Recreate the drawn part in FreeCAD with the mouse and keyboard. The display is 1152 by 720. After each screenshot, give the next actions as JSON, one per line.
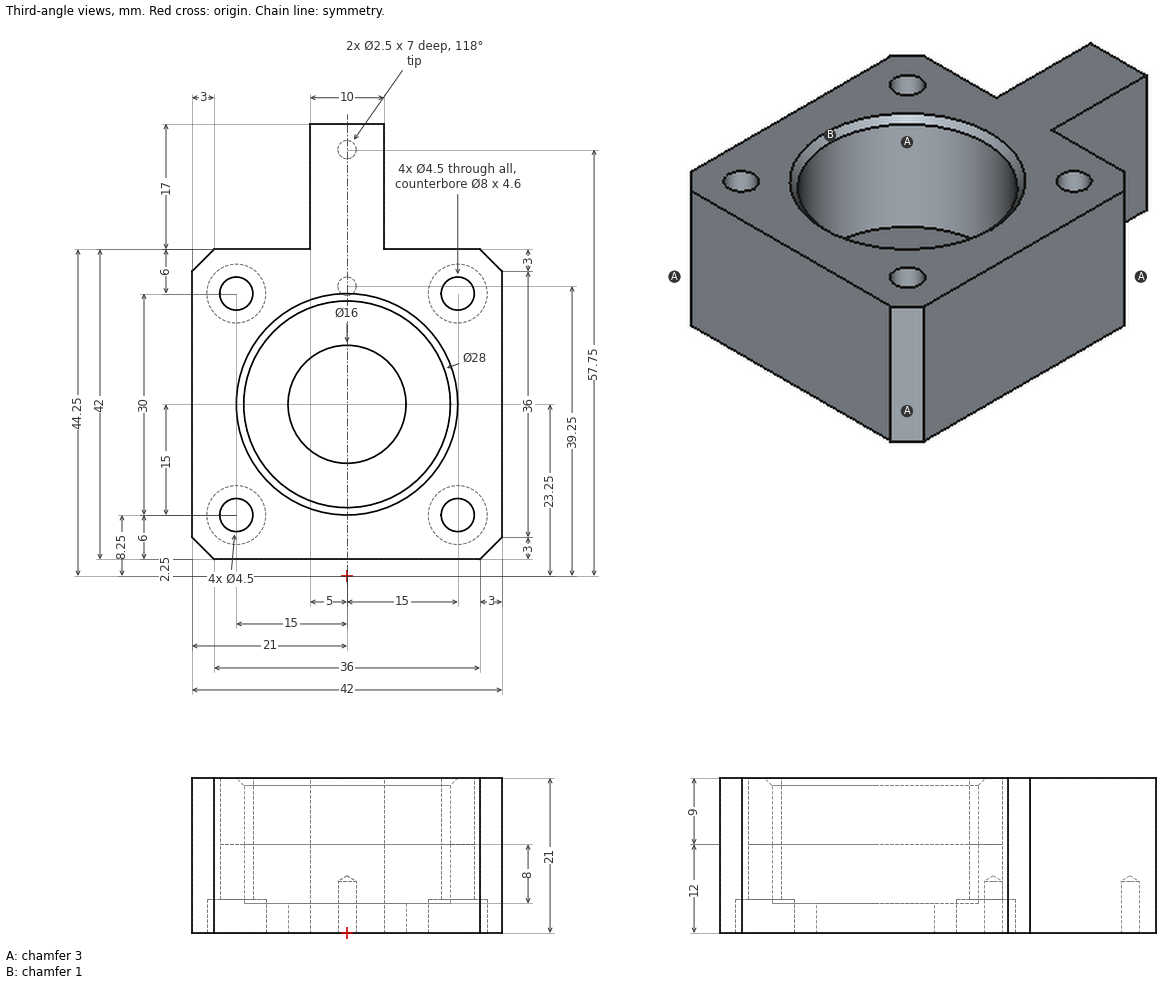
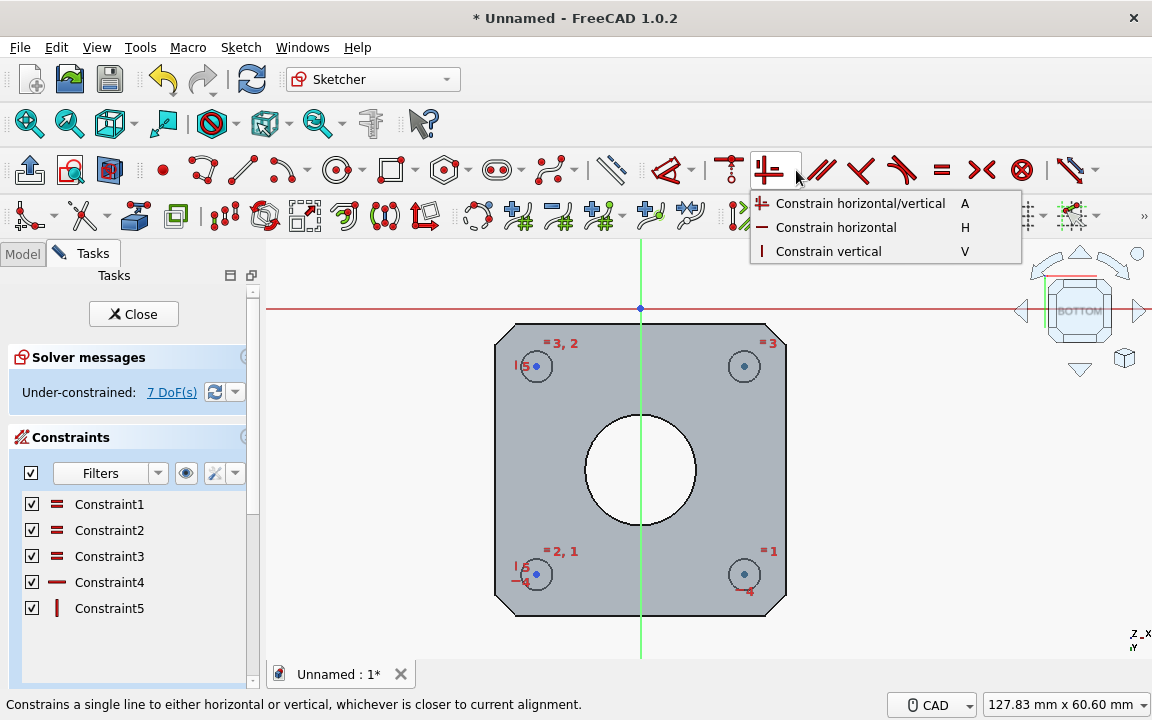
{"action": "left_click", "coordinate": [886, 251]}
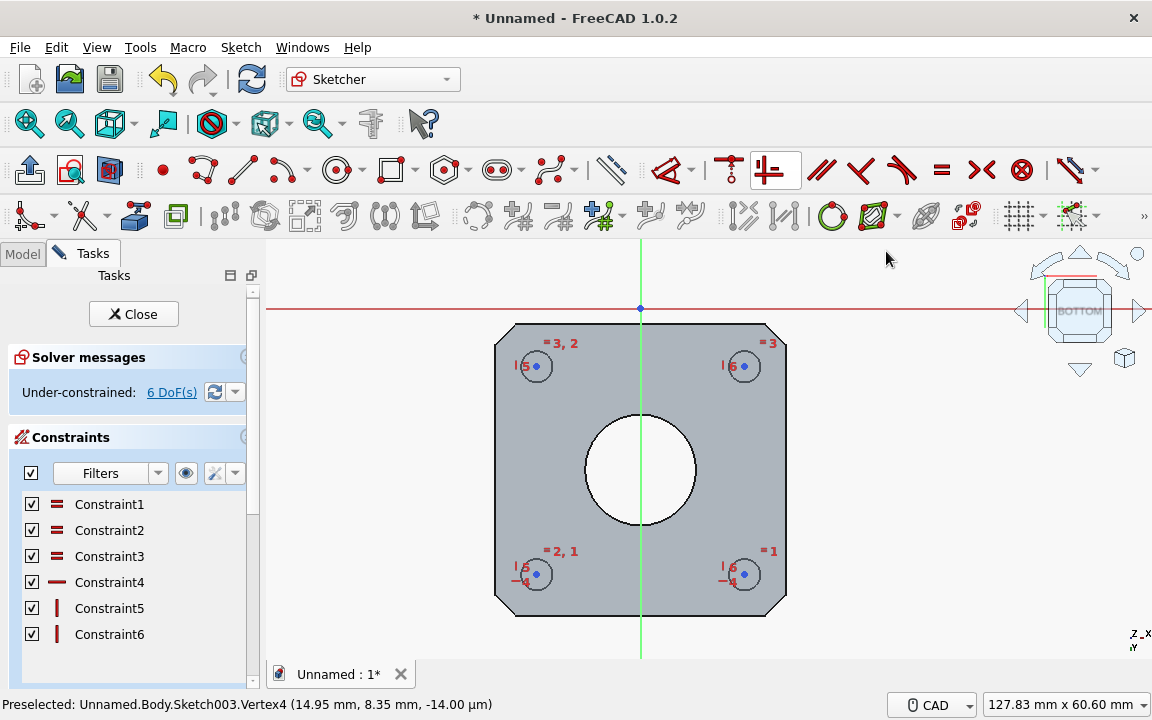
{"action": "left_click", "coordinate": [537, 367]}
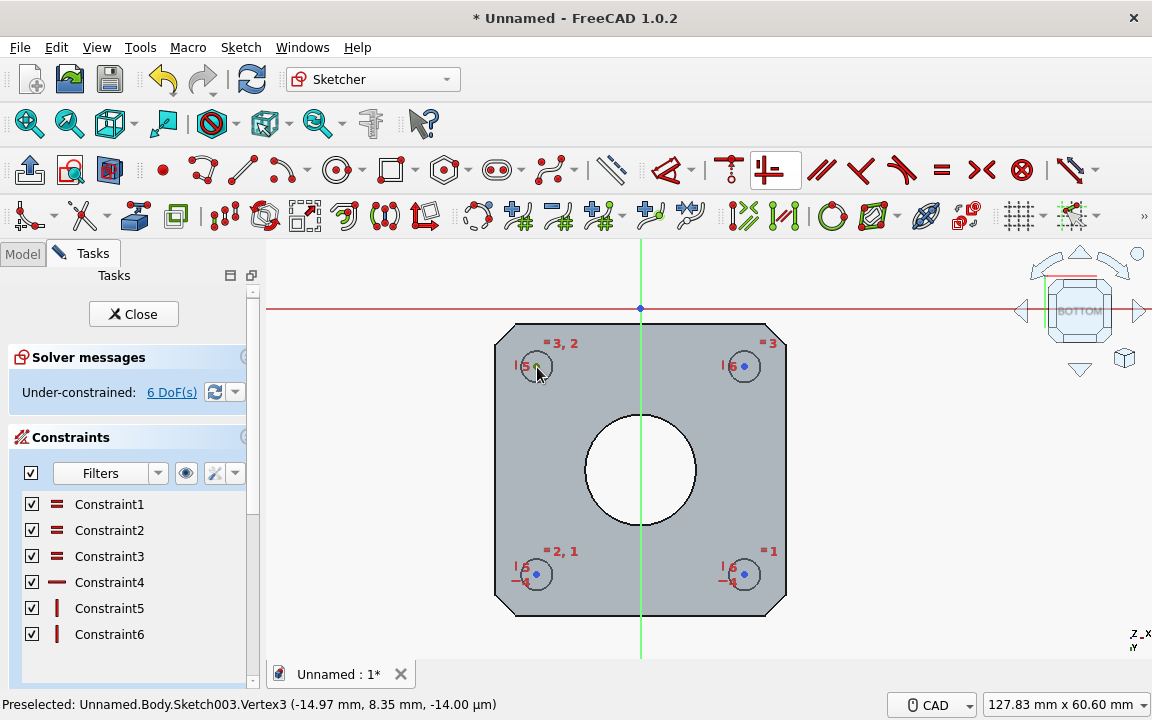
{"action": "left_click", "coordinate": [745, 367]}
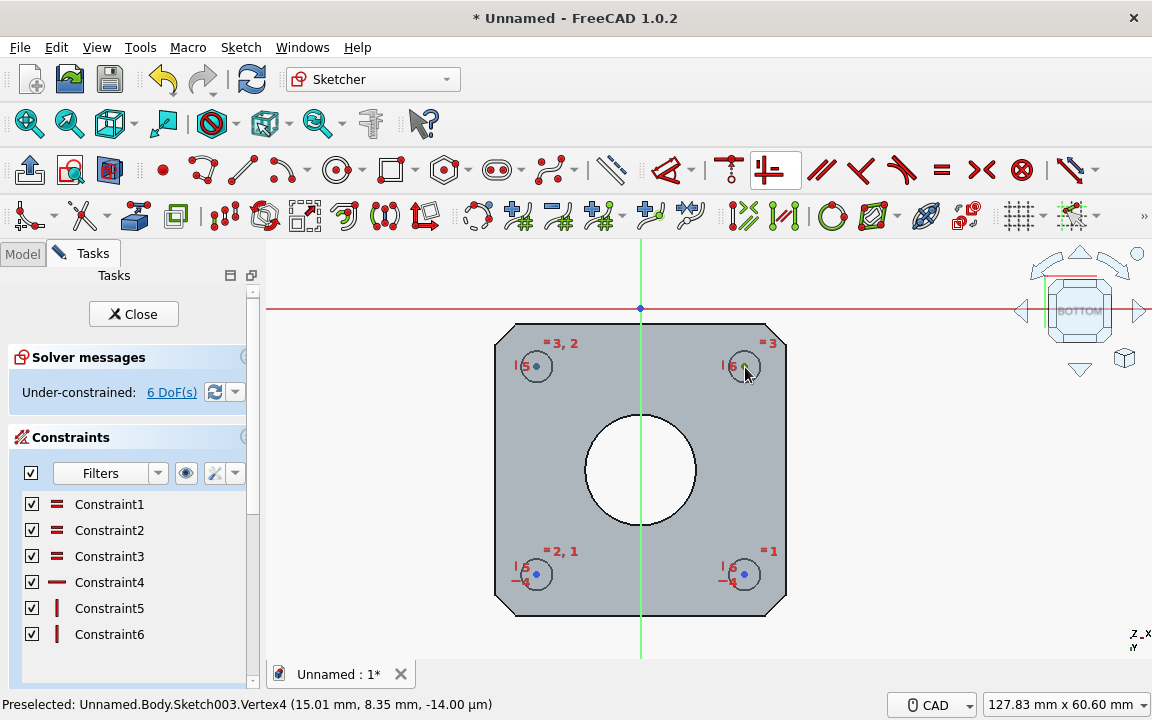
{"action": "left_click", "coordinate": [796, 170]}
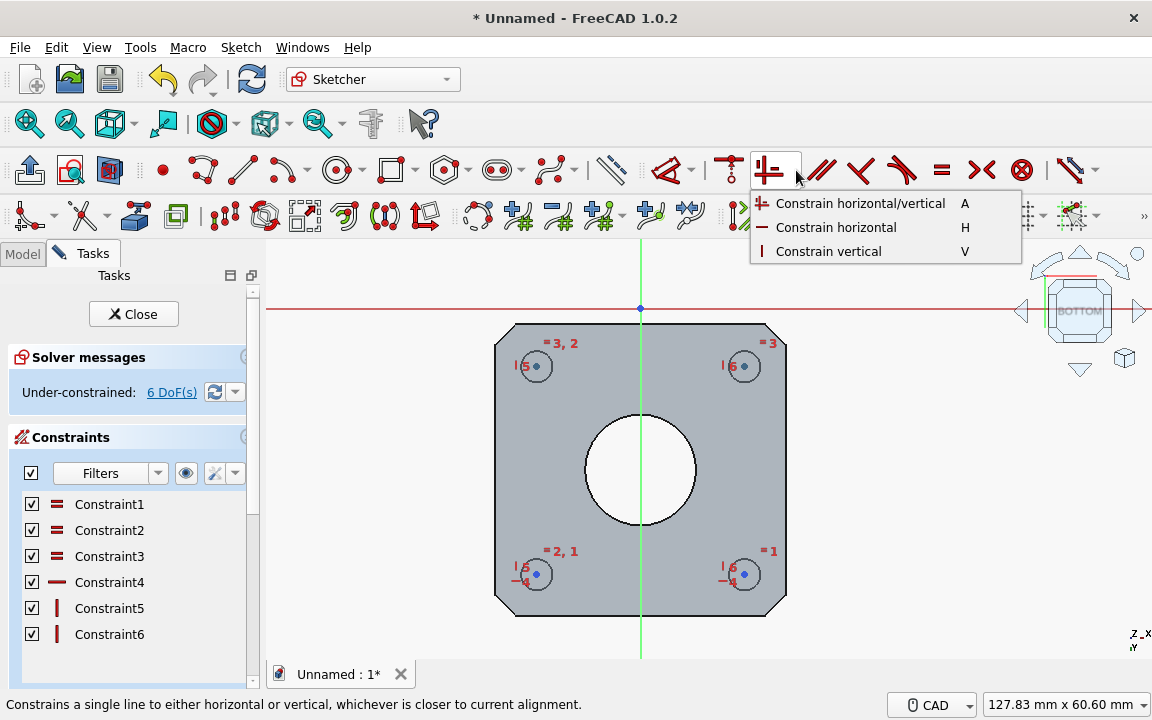
{"action": "left_click", "coordinate": [886, 227]}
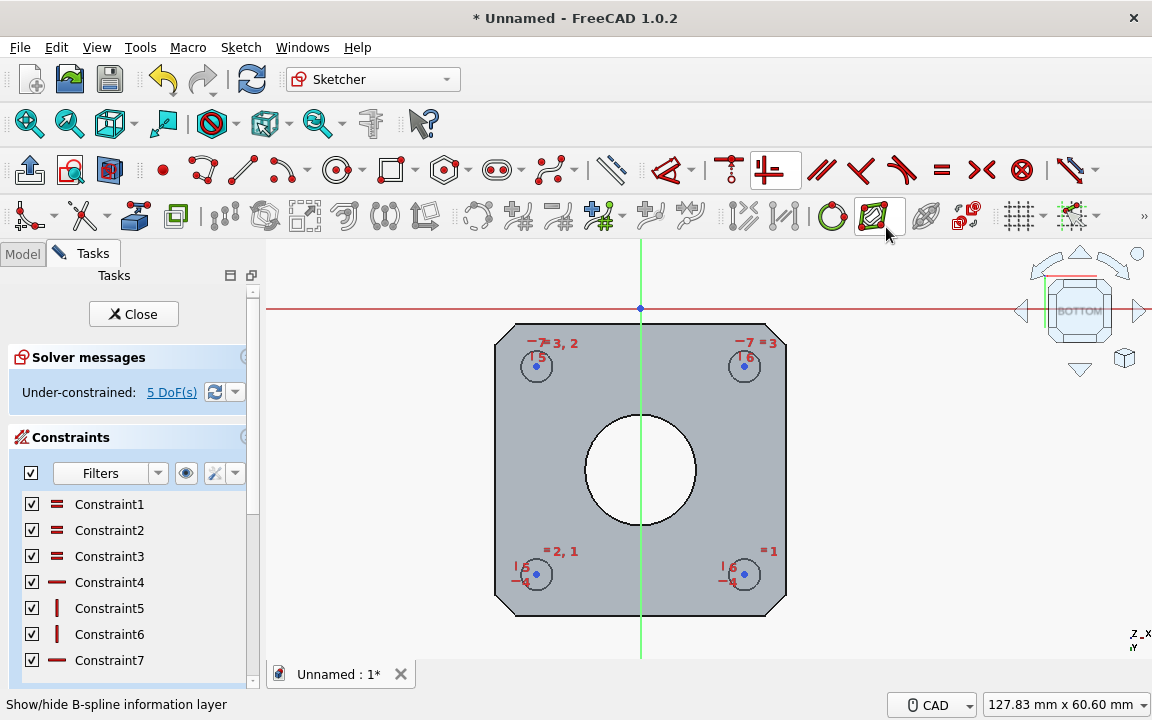
{"action": "left_click", "coordinate": [666, 170]}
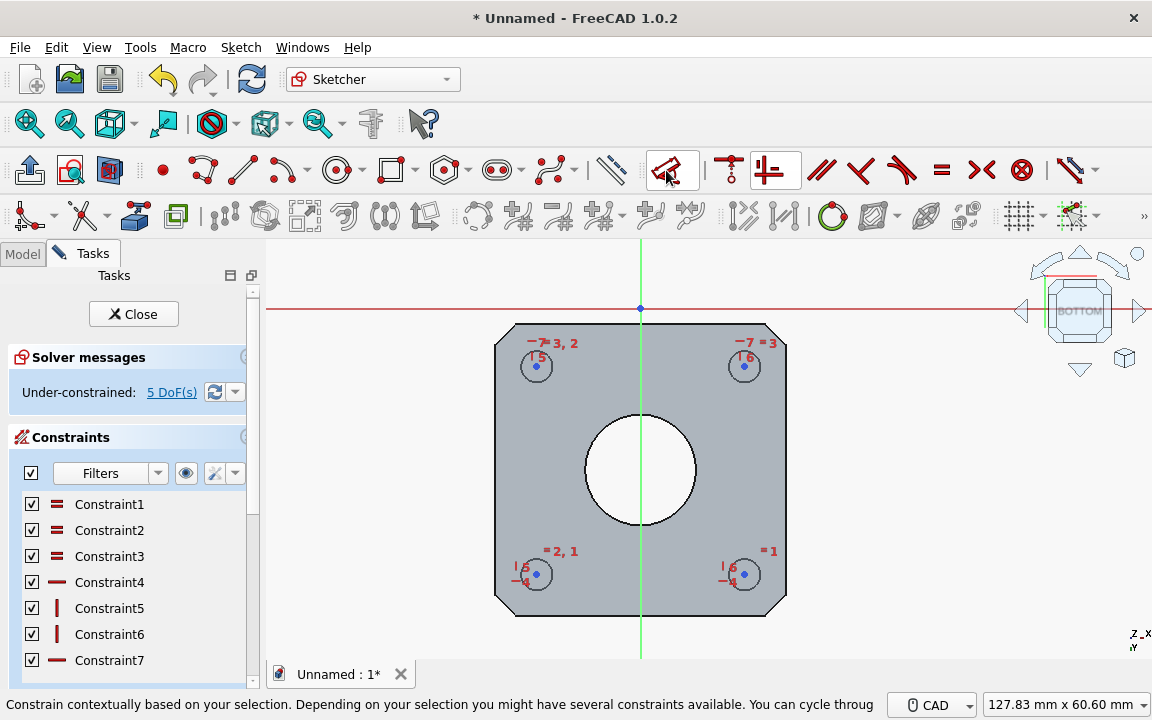
{"action": "scroll", "coordinate": [756, 564], "scroll_direction": "up", "scroll_amount": 2}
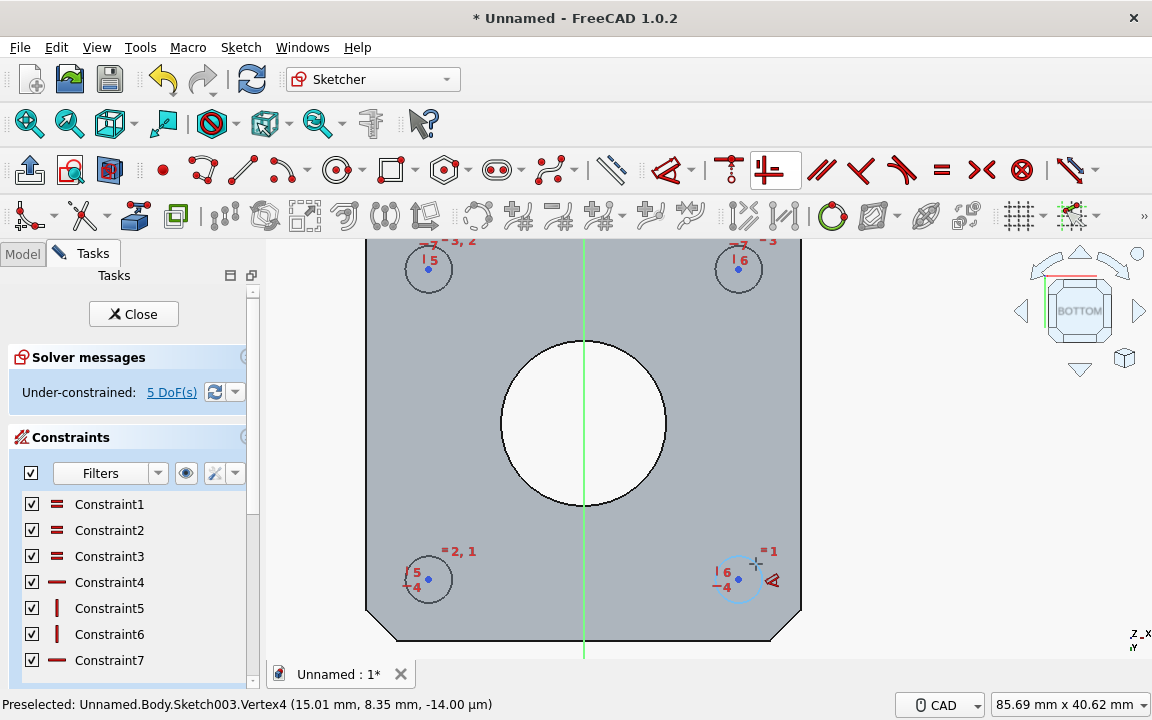
{"action": "left_click", "coordinate": [755, 563]}
{"action": "left_click", "coordinate": [777, 540]}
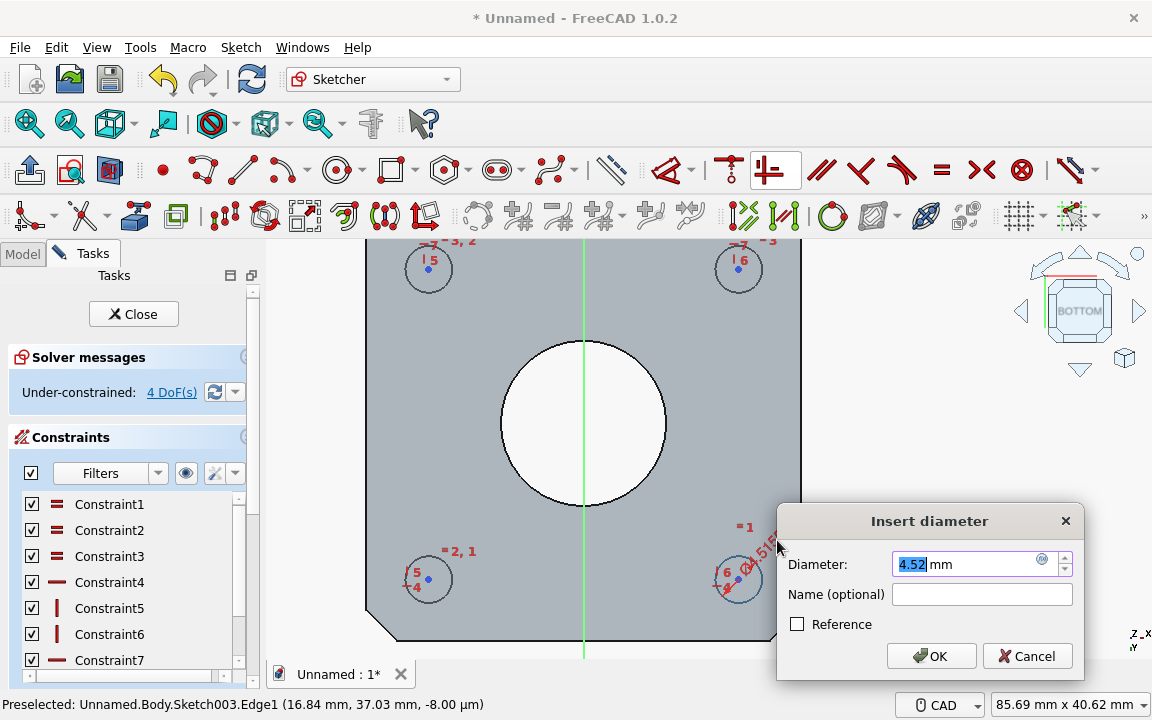
{"action": "type", "text": "4.5"}
{"action": "key", "text": "Return"}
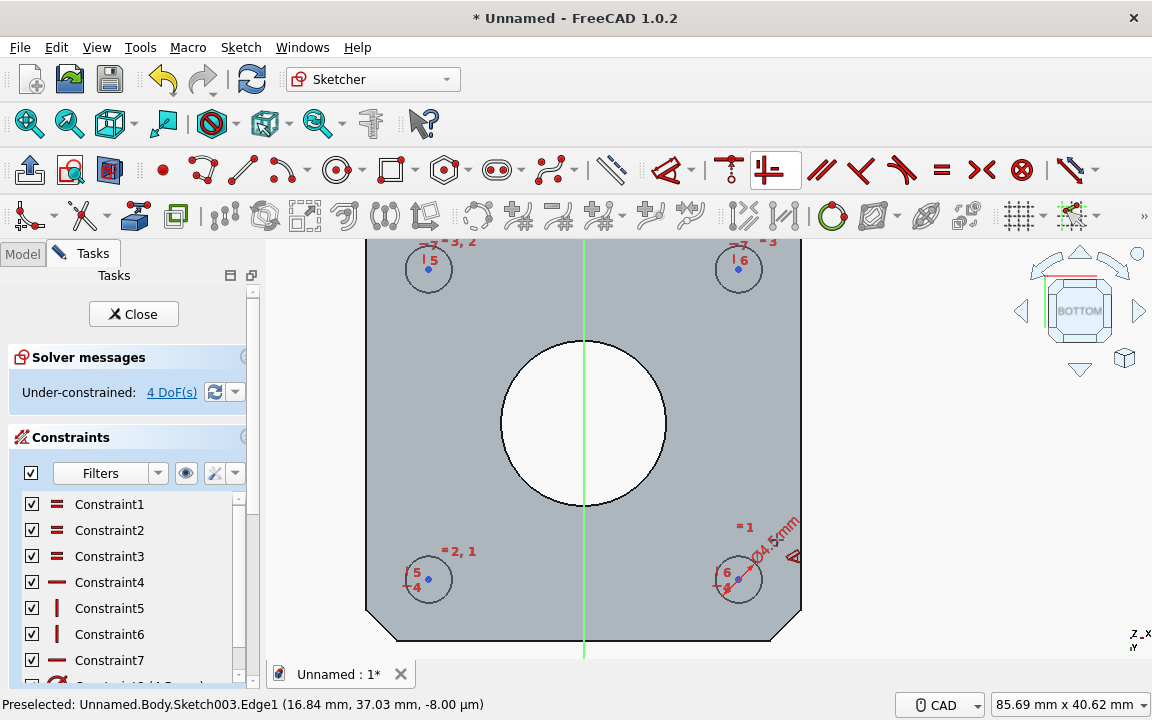
{"action": "left_click", "coordinate": [739, 580]}
{"action": "left_click", "coordinate": [661, 614]}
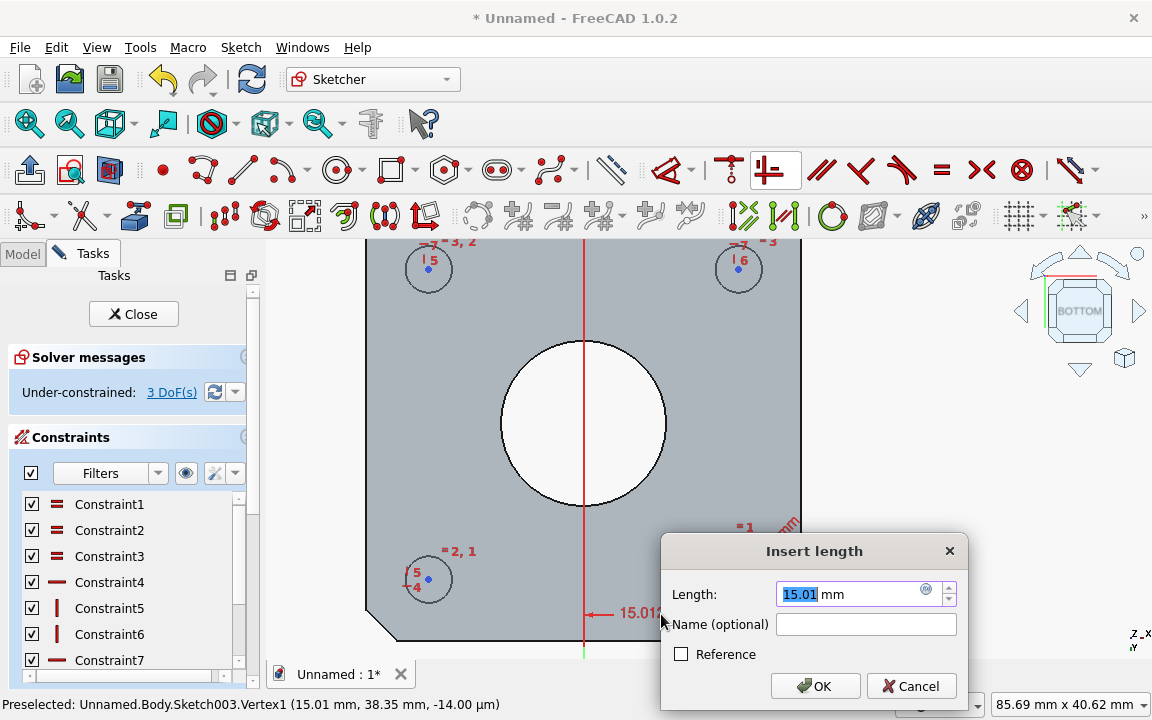
{"action": "type", "text": "15"}
{"action": "key", "text": "Return"}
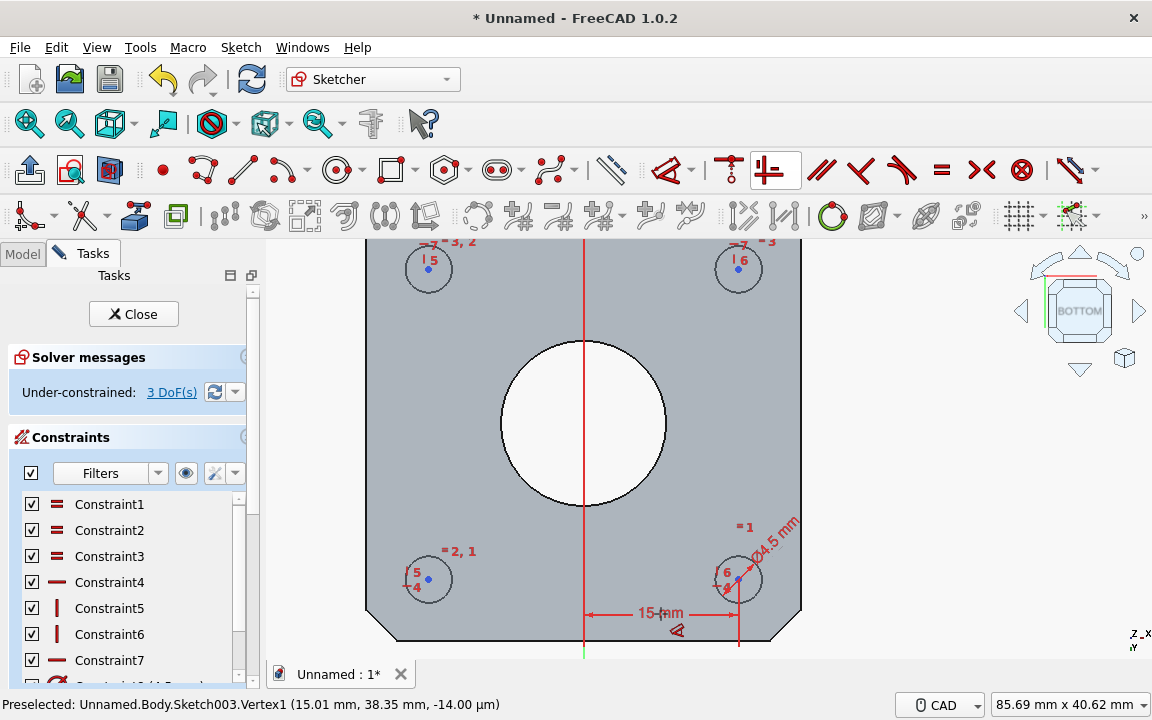
{"action": "left_click", "coordinate": [429, 580]}
{"action": "left_click", "coordinate": [506, 614]}